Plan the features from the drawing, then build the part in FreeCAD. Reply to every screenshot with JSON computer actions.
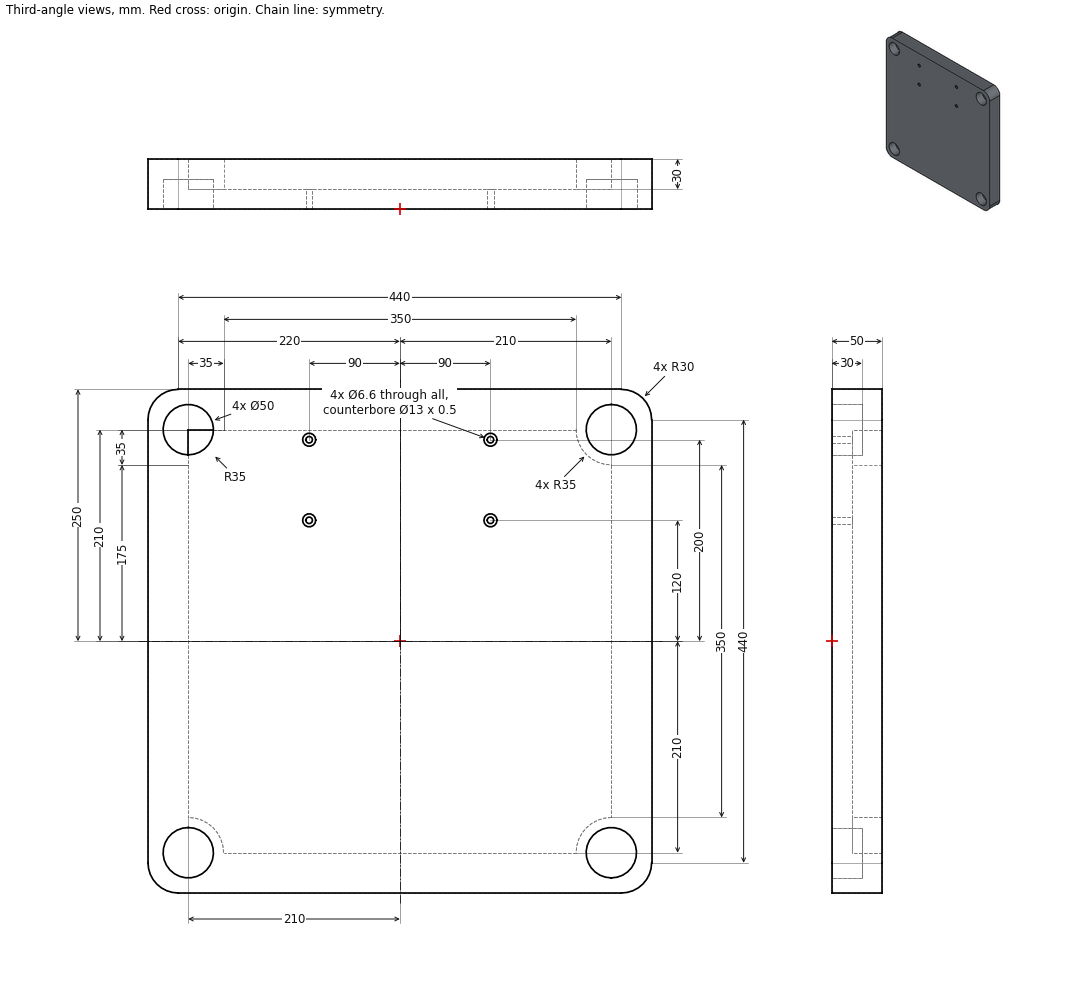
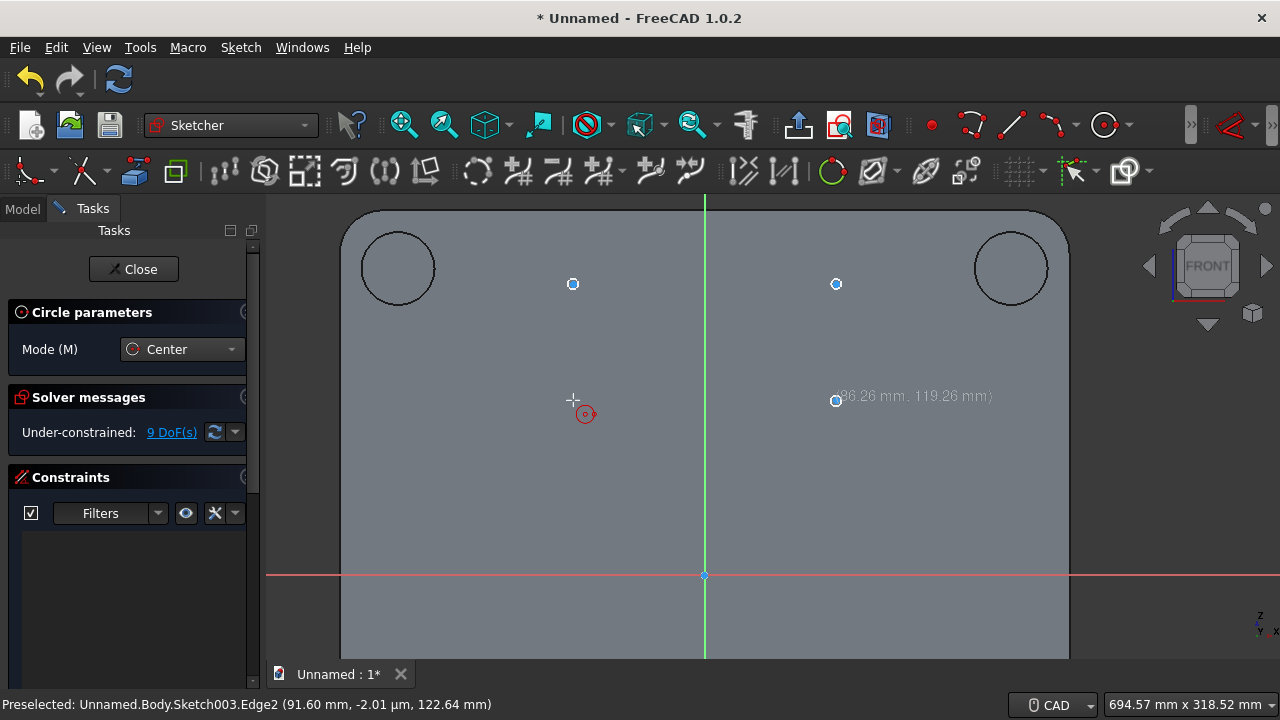
{"action": "left_click", "coordinate": [573, 400]}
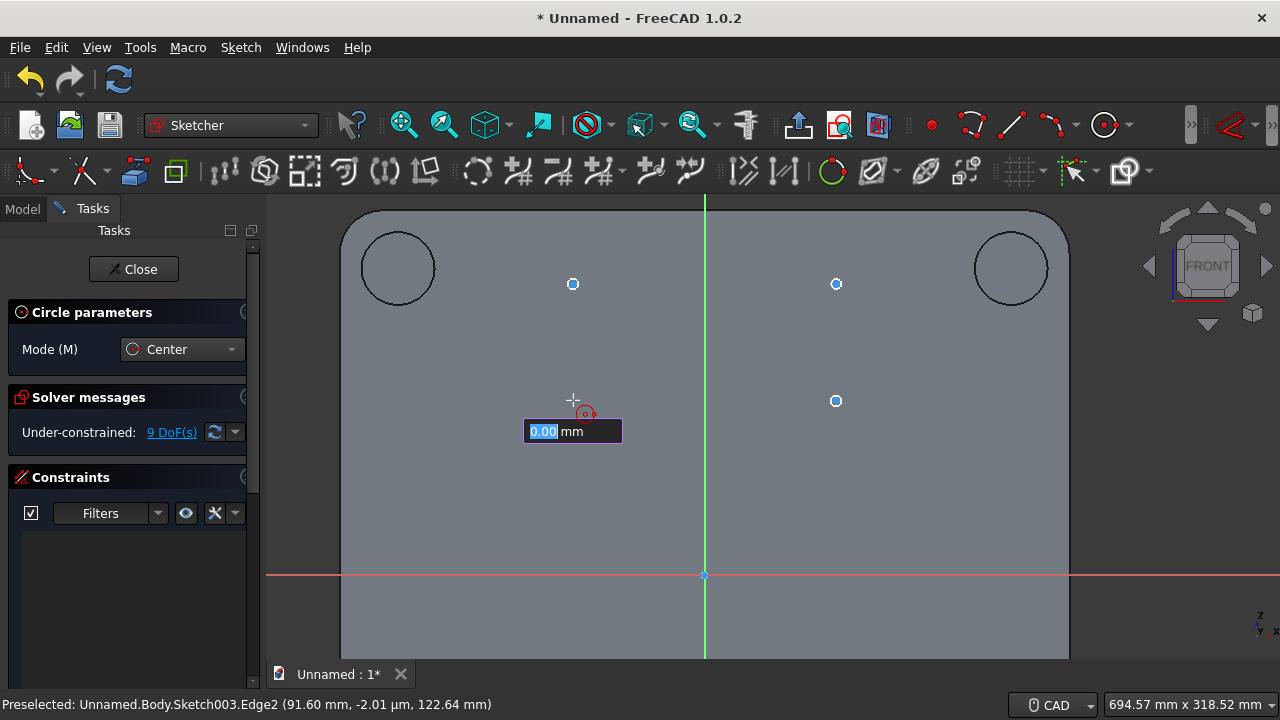
{"action": "scroll", "coordinate": [577, 397], "scroll_direction": "up", "scroll_amount": 6}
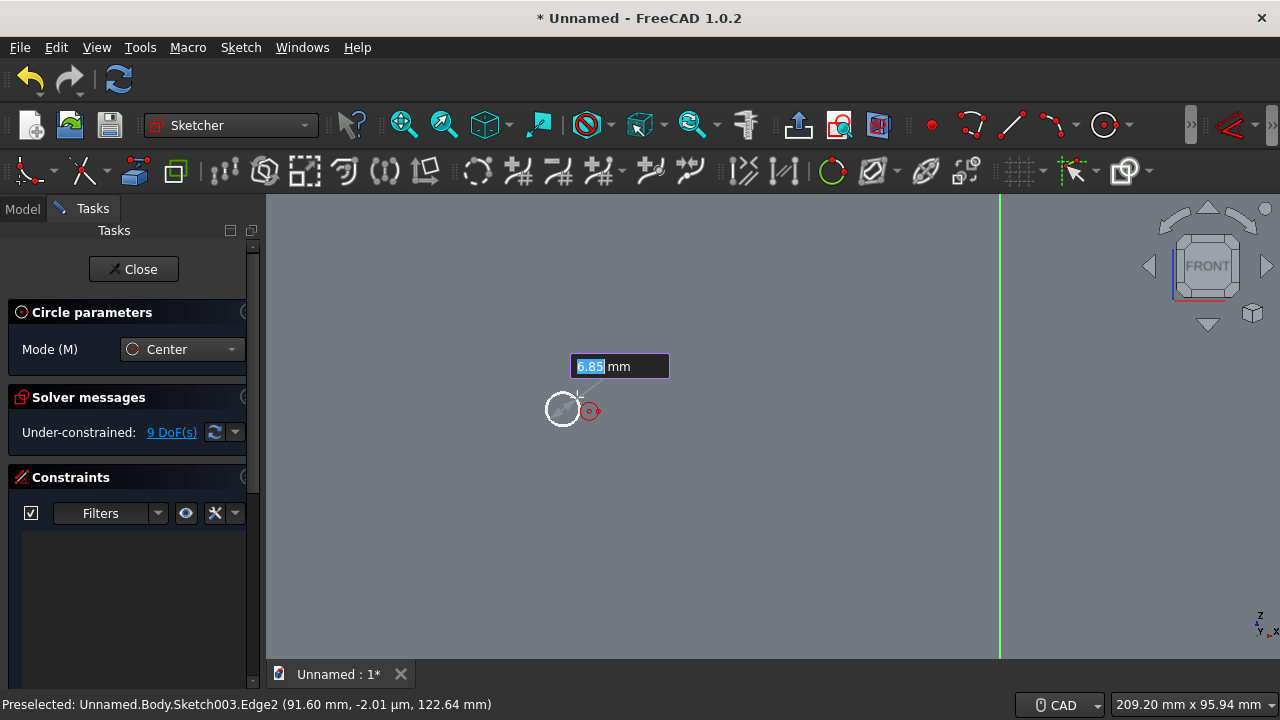
{"action": "left_click", "coordinate": [575, 394]}
{"action": "key", "text": "Escape"}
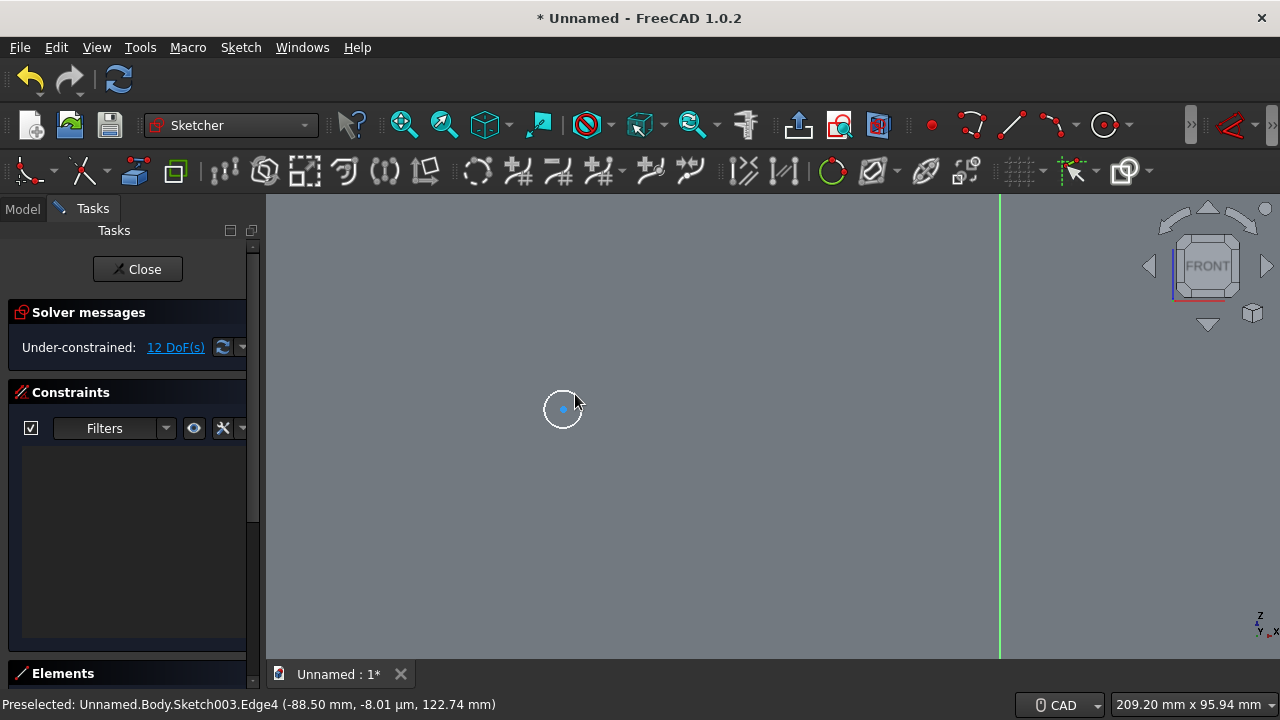
{"action": "scroll", "coordinate": [577, 397], "scroll_direction": "down", "scroll_amount": 6}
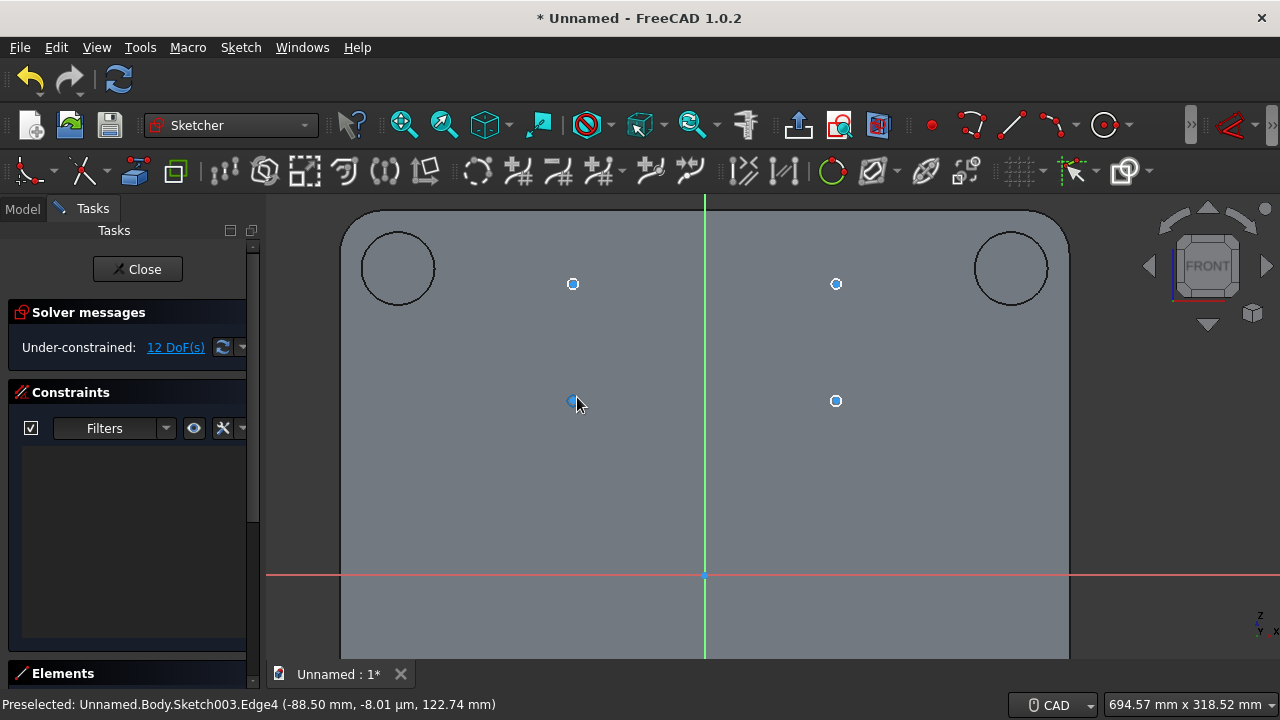
{"action": "scroll", "coordinate": [840, 280], "scroll_direction": "up", "scroll_amount": 6}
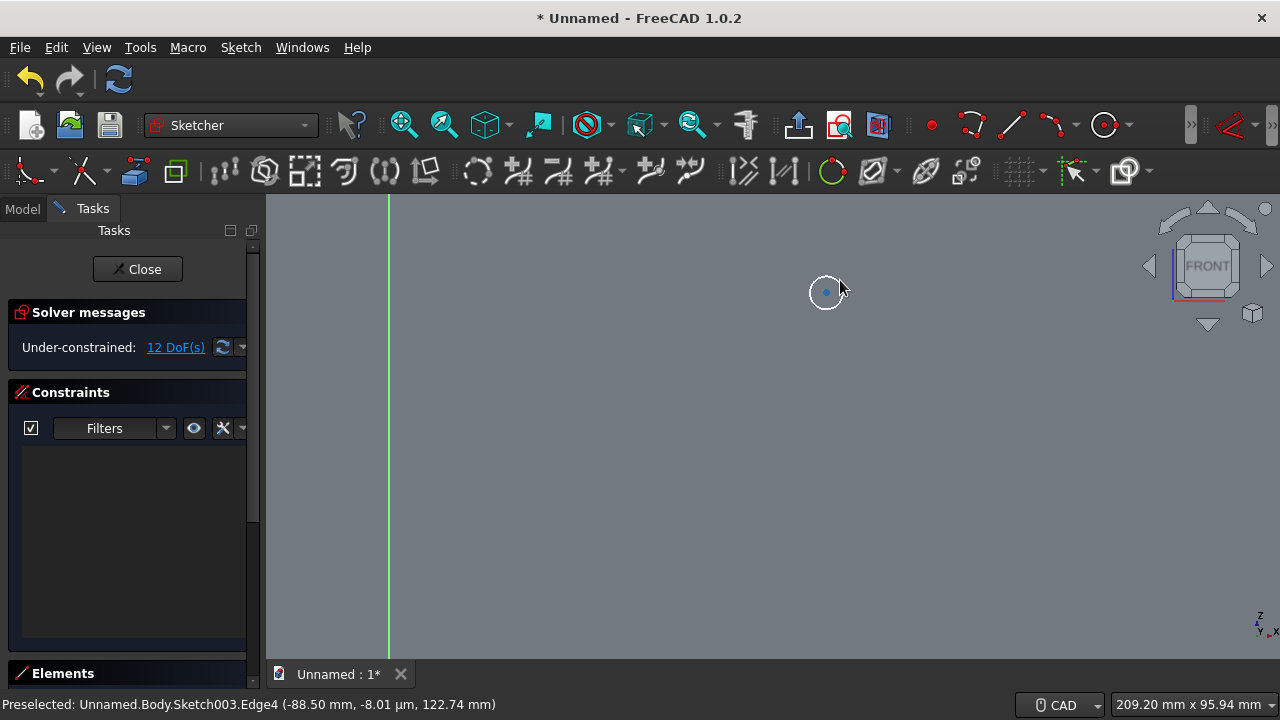
{"action": "left_click", "coordinate": [838, 281]}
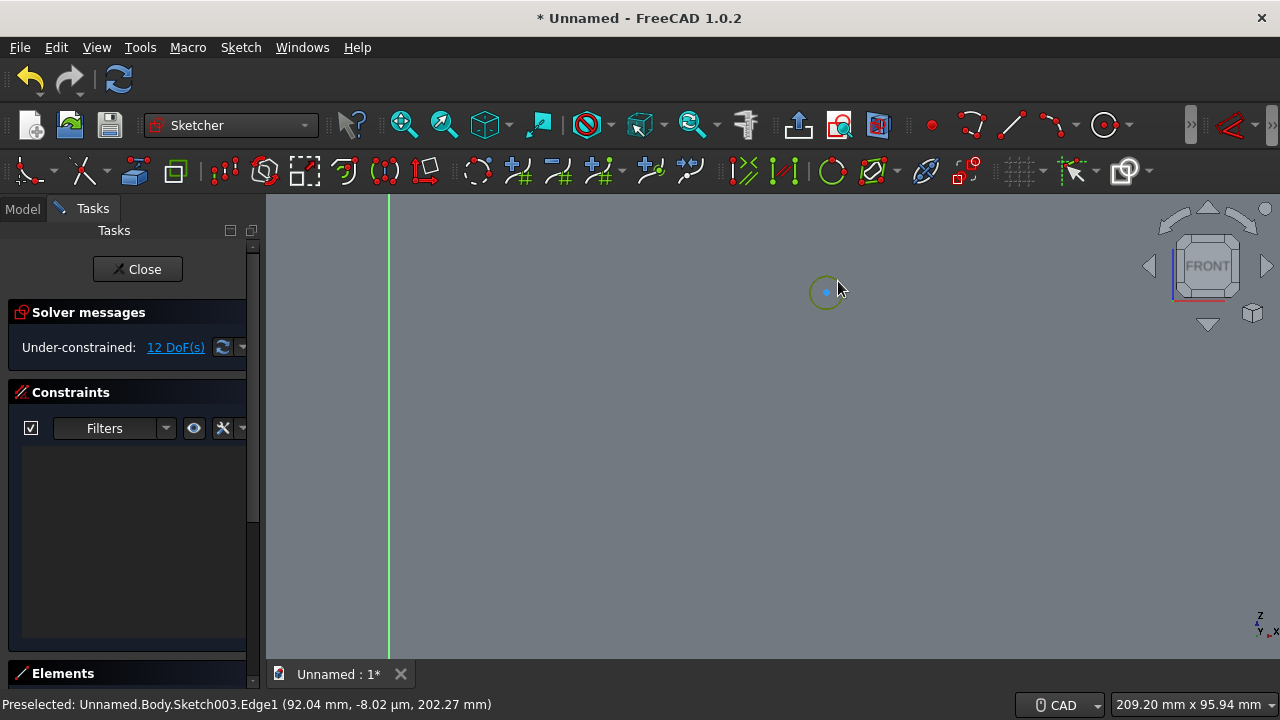
{"action": "scroll", "coordinate": [840, 280], "scroll_direction": "down", "scroll_amount": 6}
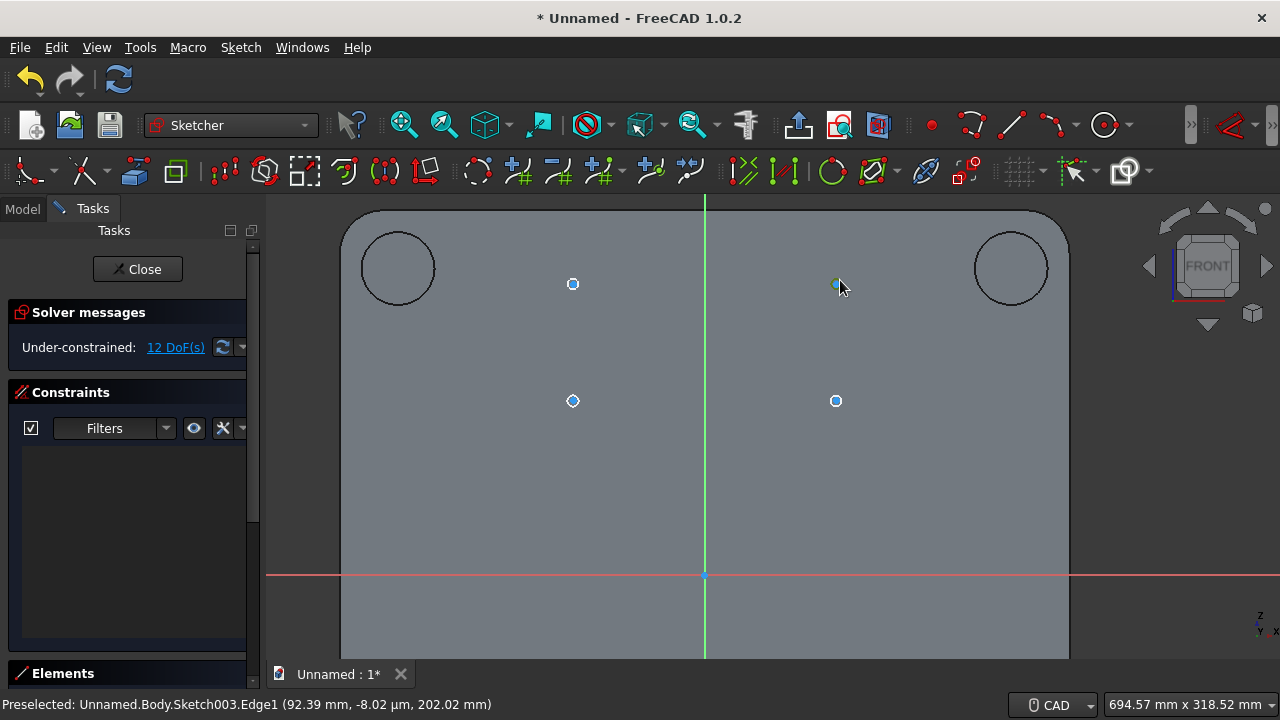
{"action": "scroll", "coordinate": [577, 280], "scroll_direction": "up", "scroll_amount": 5}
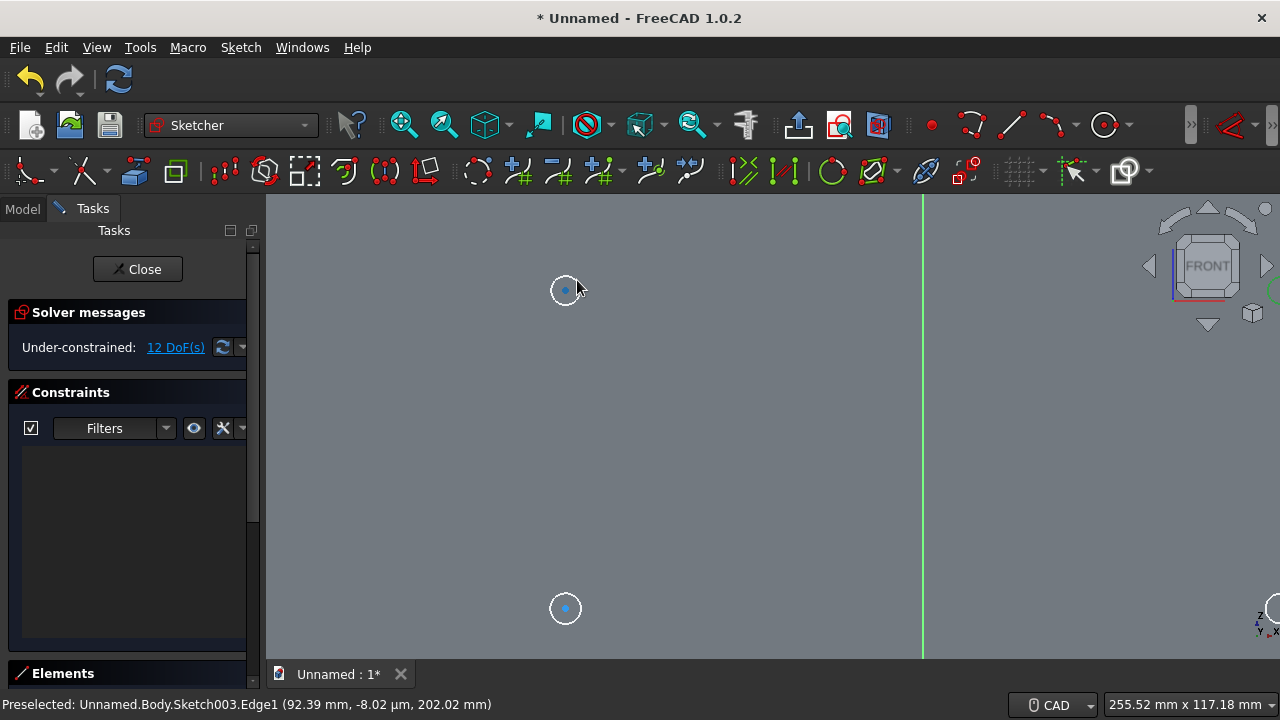
{"action": "left_click", "coordinate": [576, 280]}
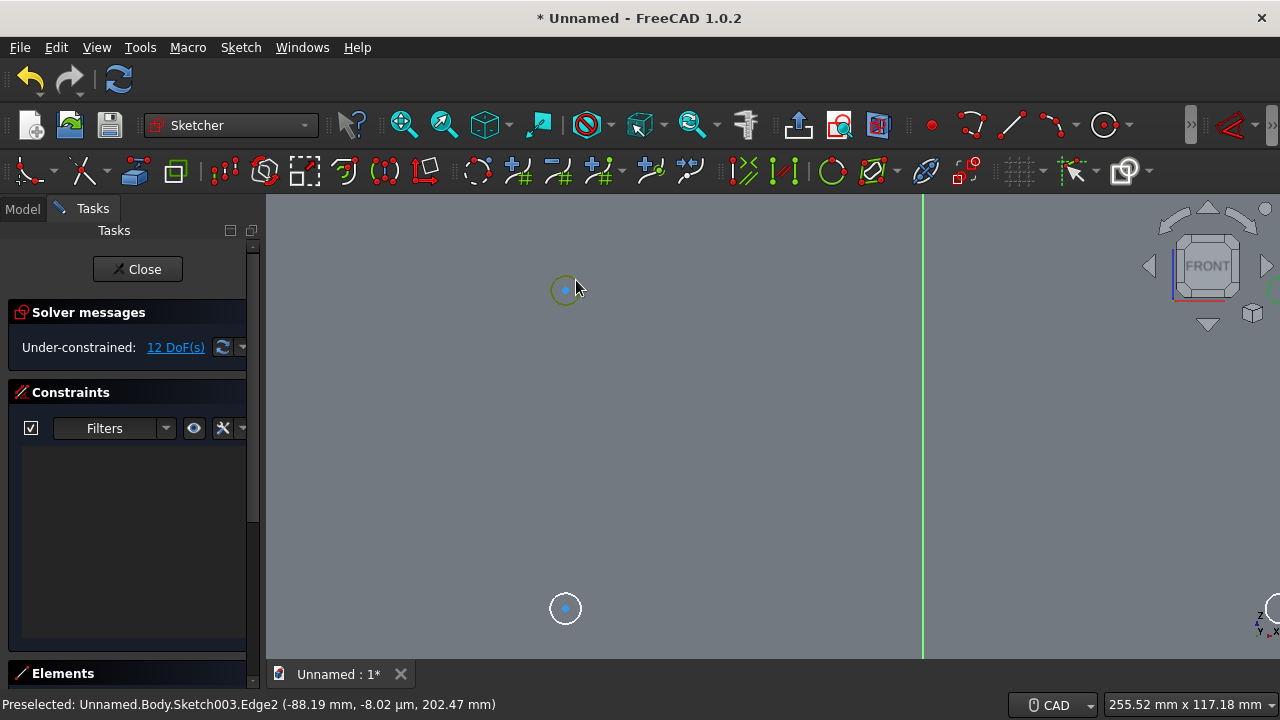
{"action": "scroll", "coordinate": [577, 280], "scroll_direction": "down", "scroll_amount": 5}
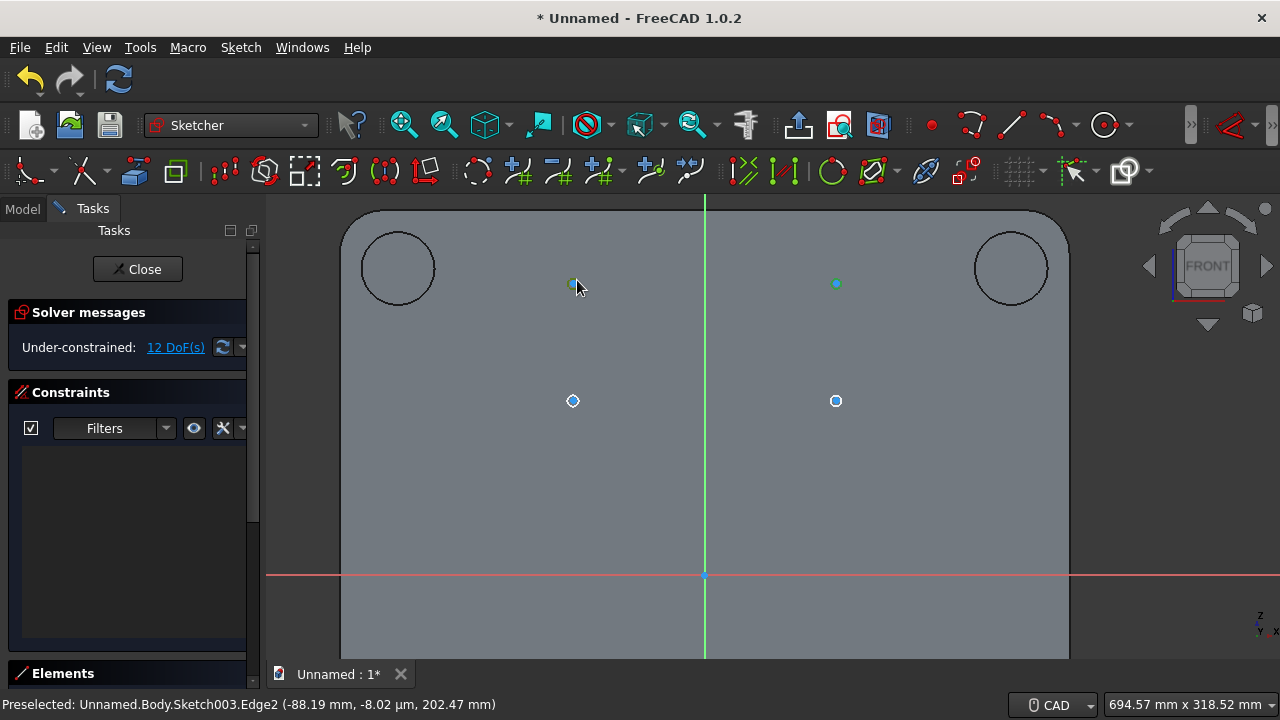
{"action": "scroll", "coordinate": [840, 397], "scroll_direction": "up", "scroll_amount": 5}